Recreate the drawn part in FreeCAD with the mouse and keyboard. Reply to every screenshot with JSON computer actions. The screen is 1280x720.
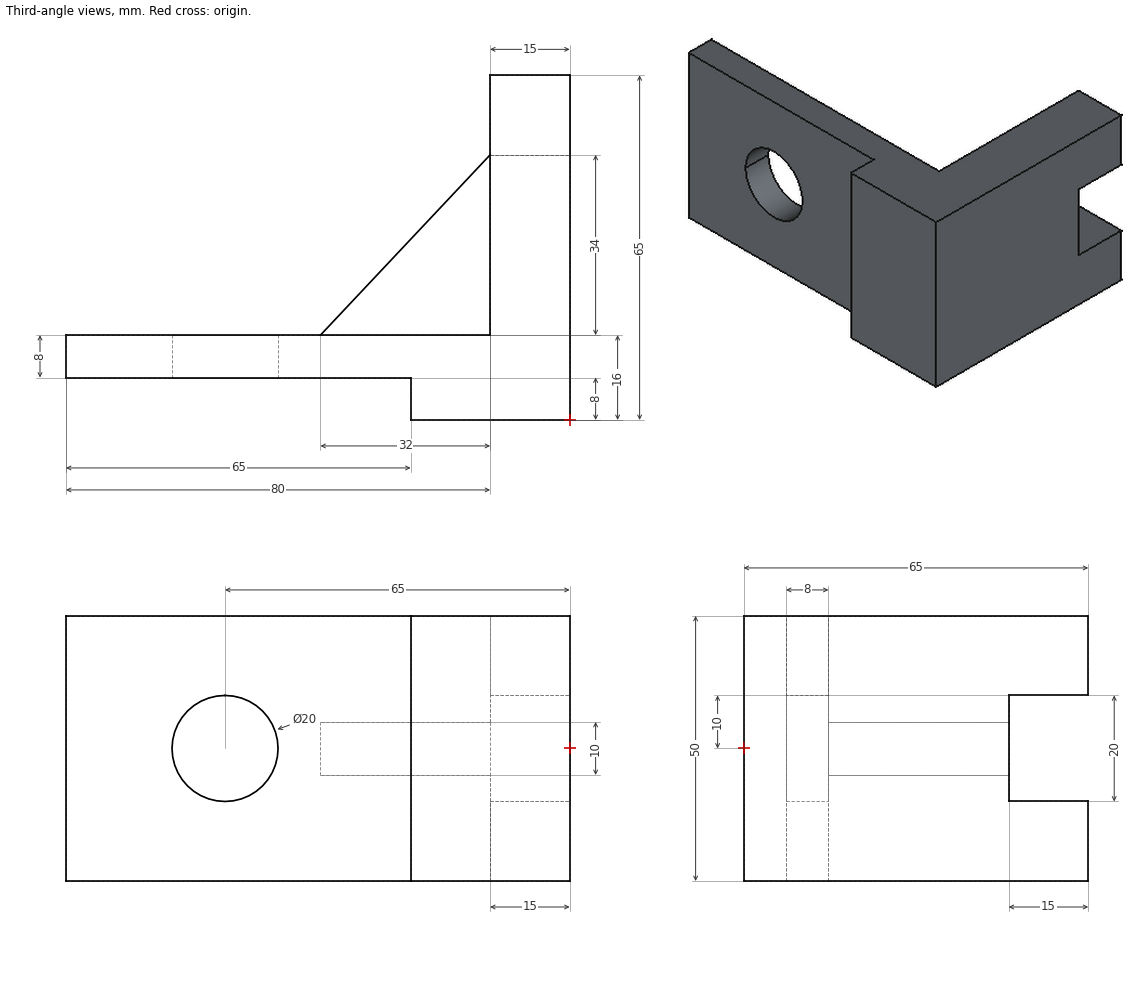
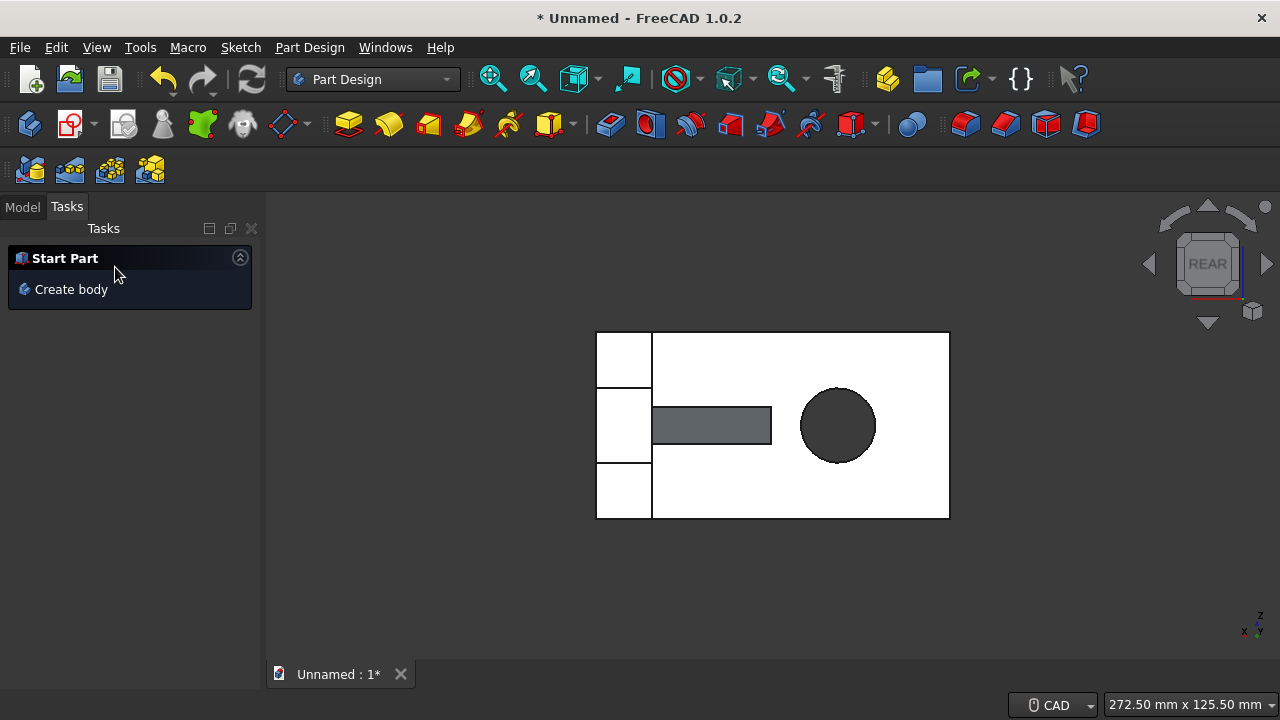
{"action": "key", "text": "0"}